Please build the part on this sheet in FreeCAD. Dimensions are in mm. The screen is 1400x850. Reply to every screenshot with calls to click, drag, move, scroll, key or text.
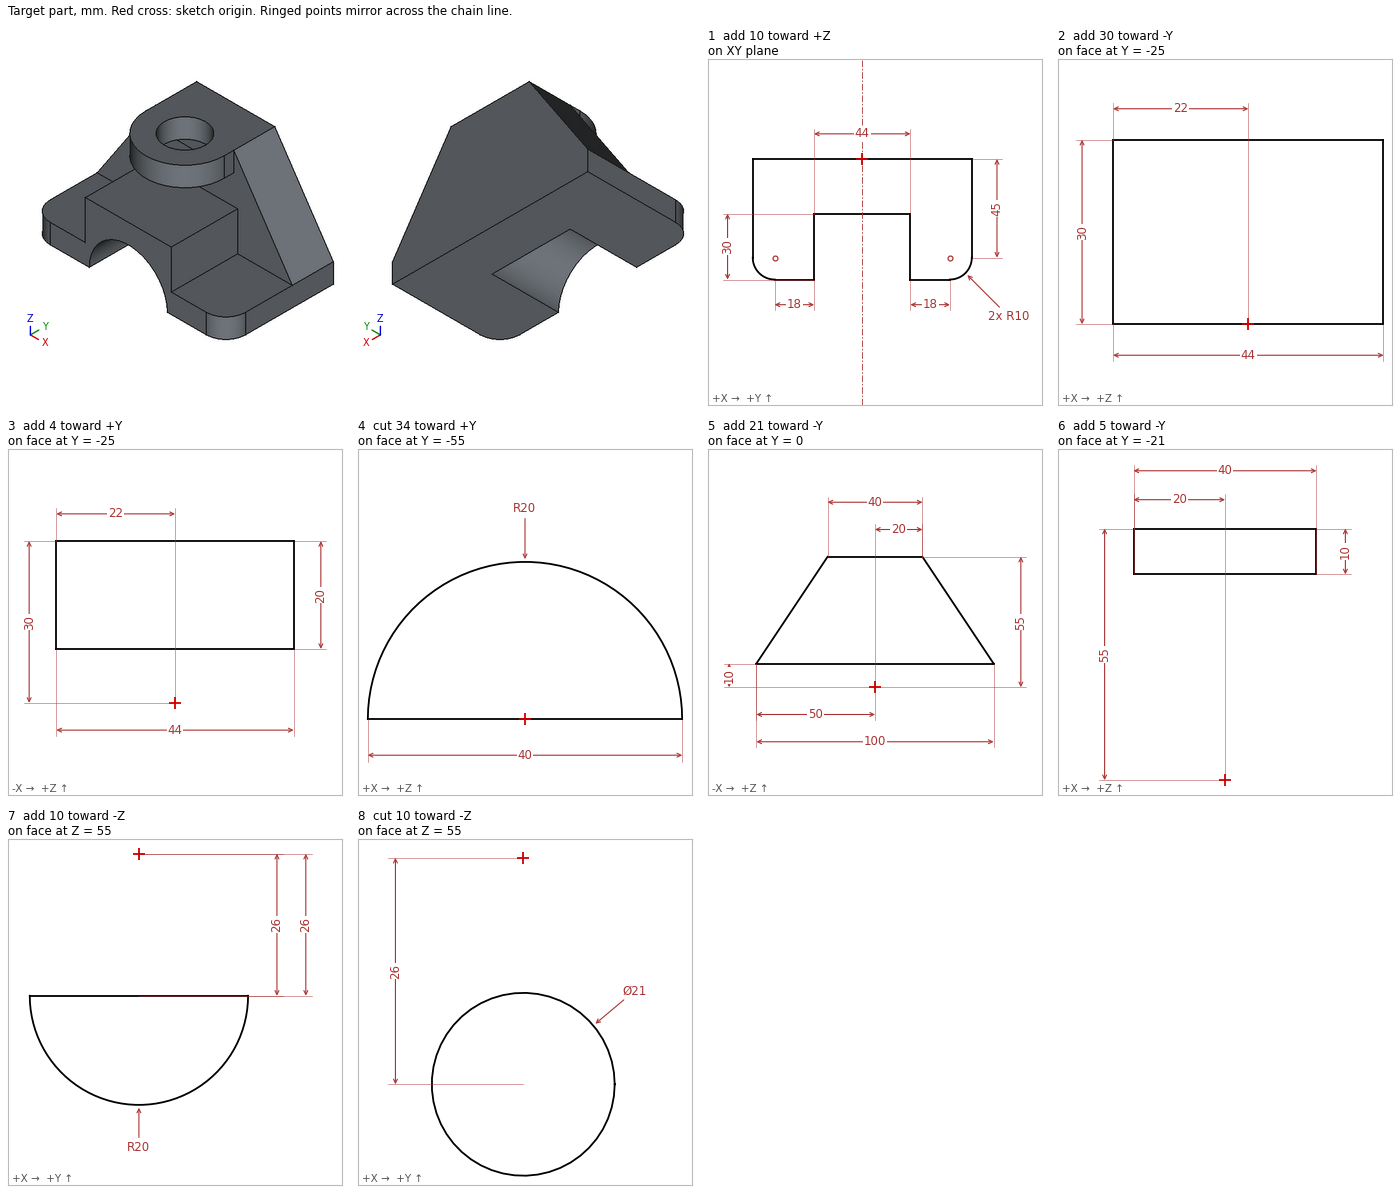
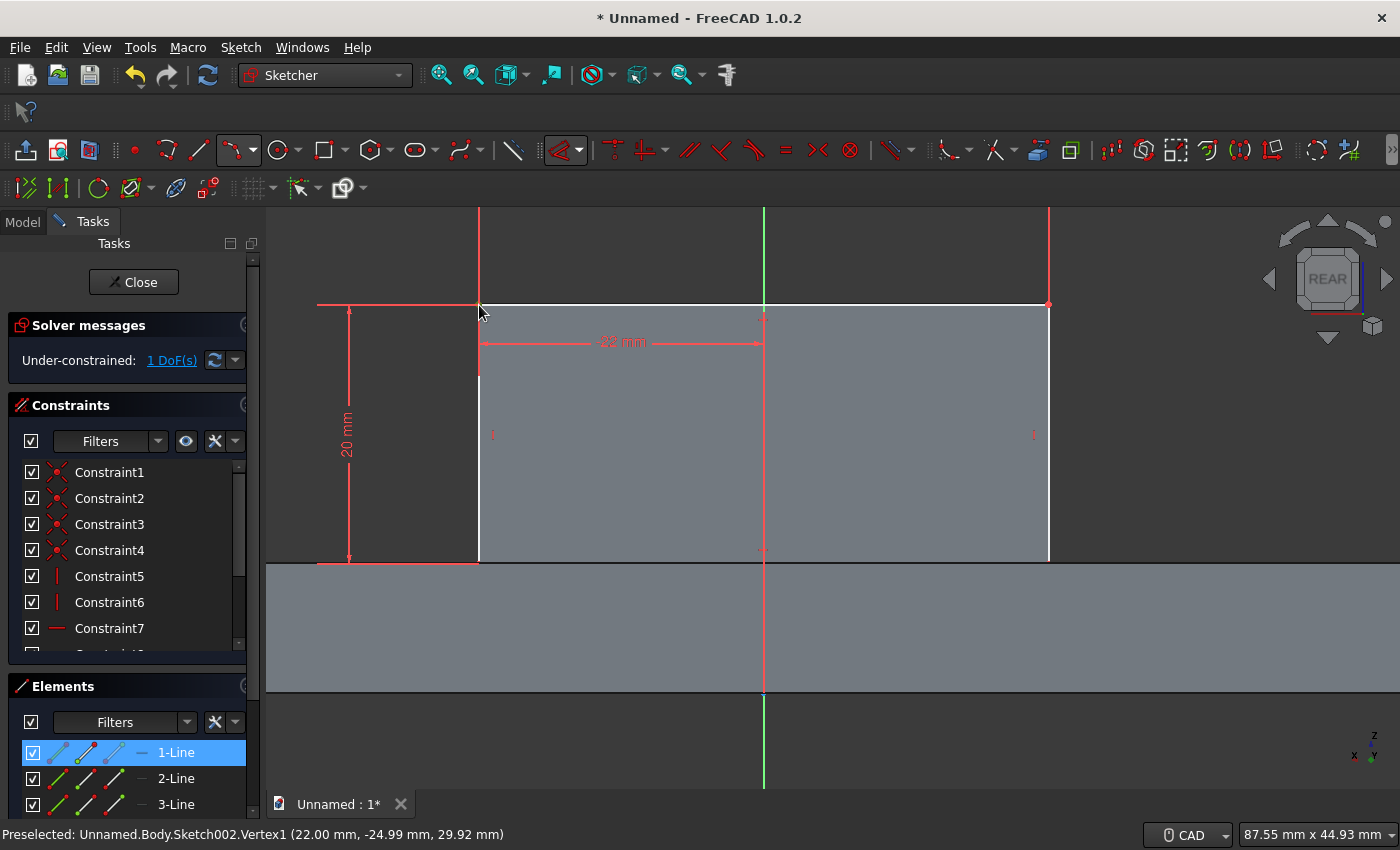
click(582, 150)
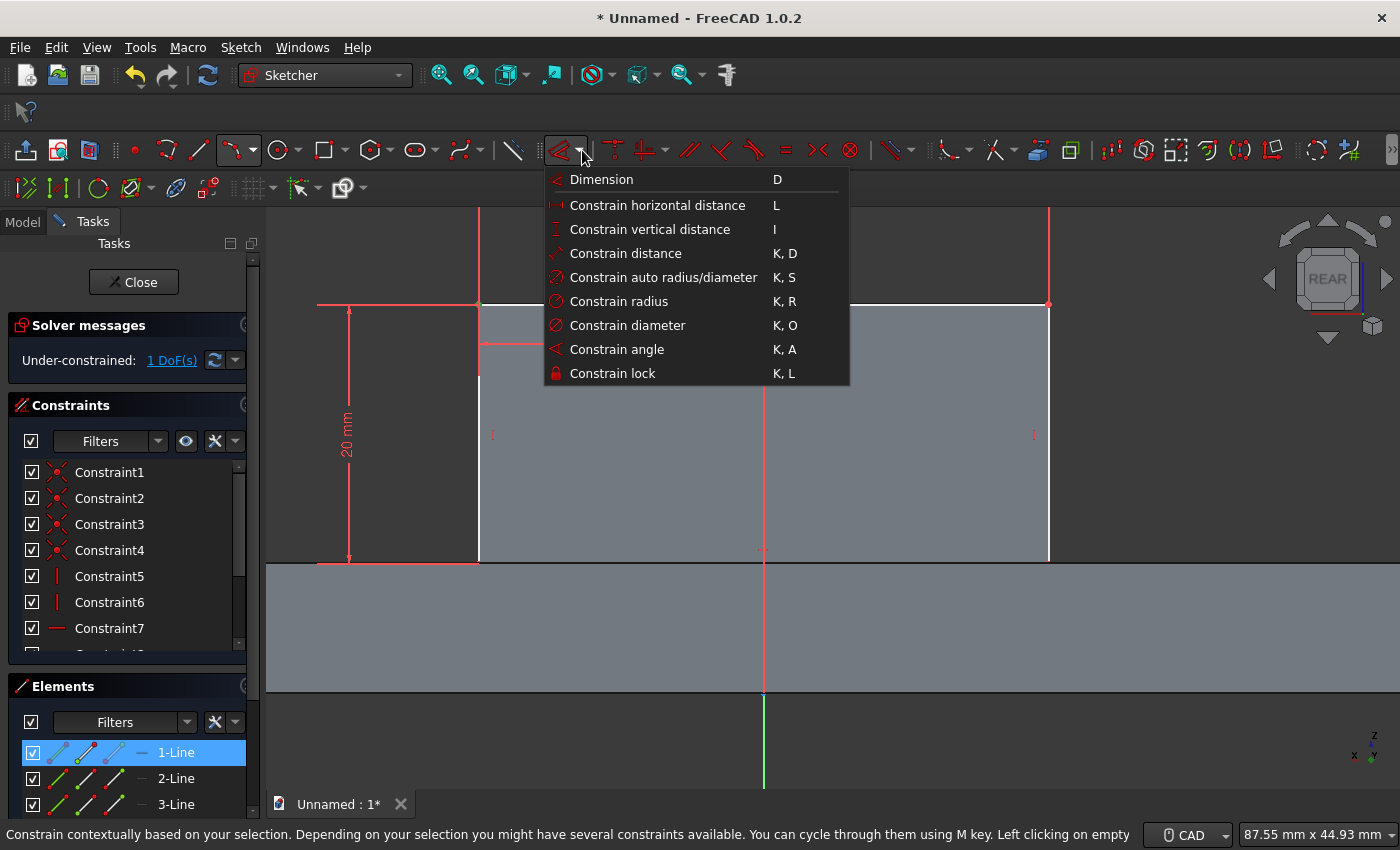
click(697, 229)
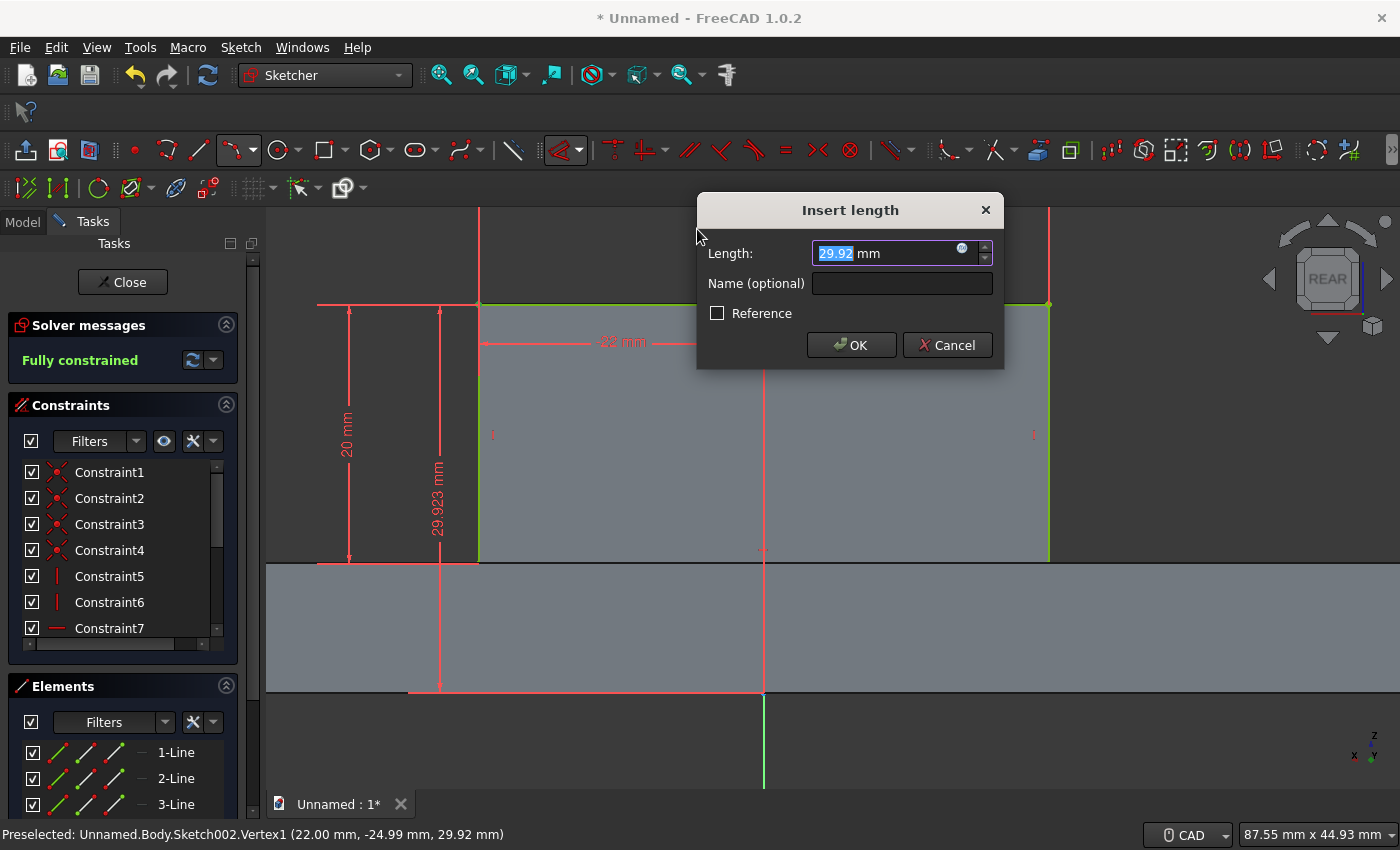
text(30)
key(Return)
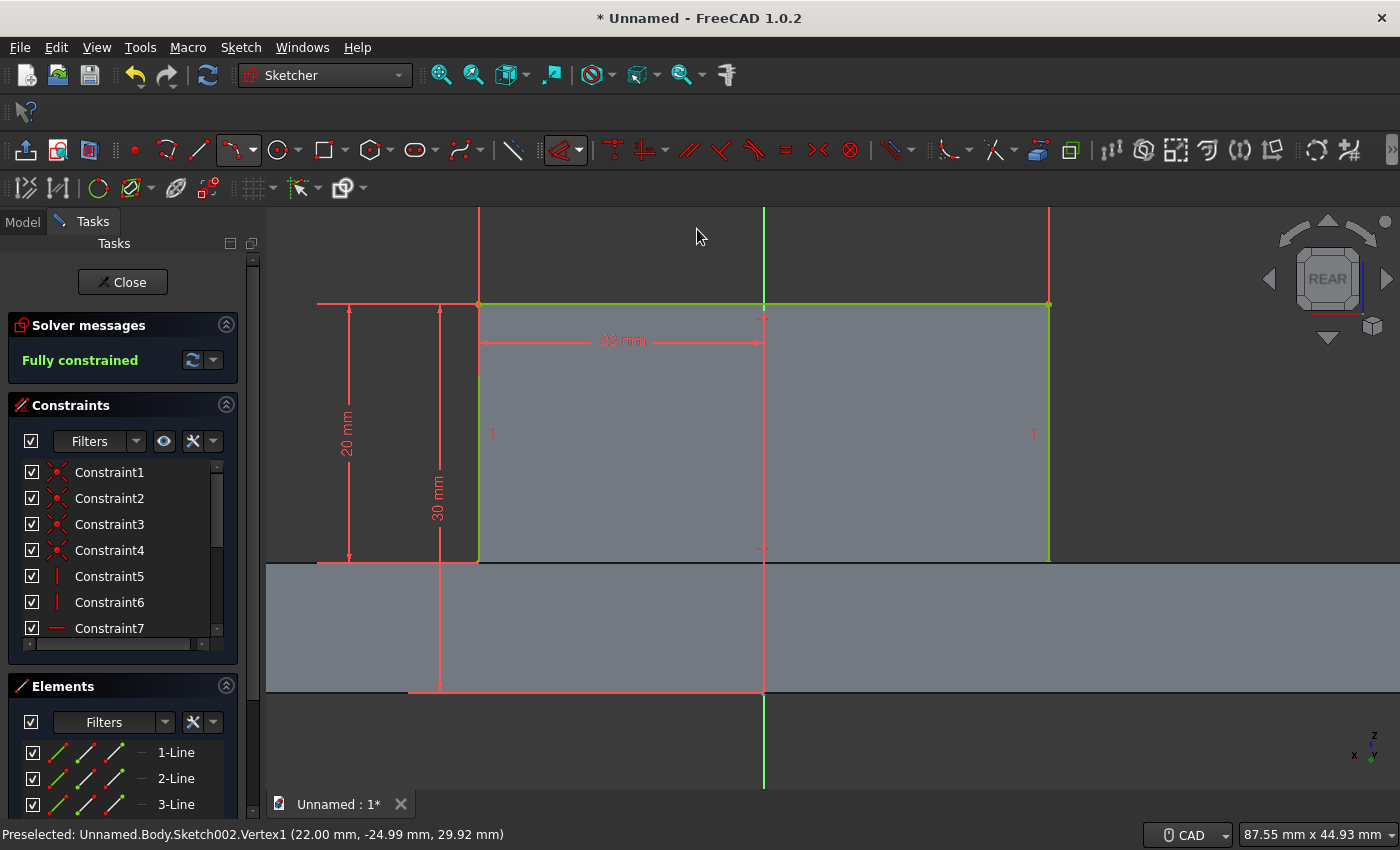
click(123, 282)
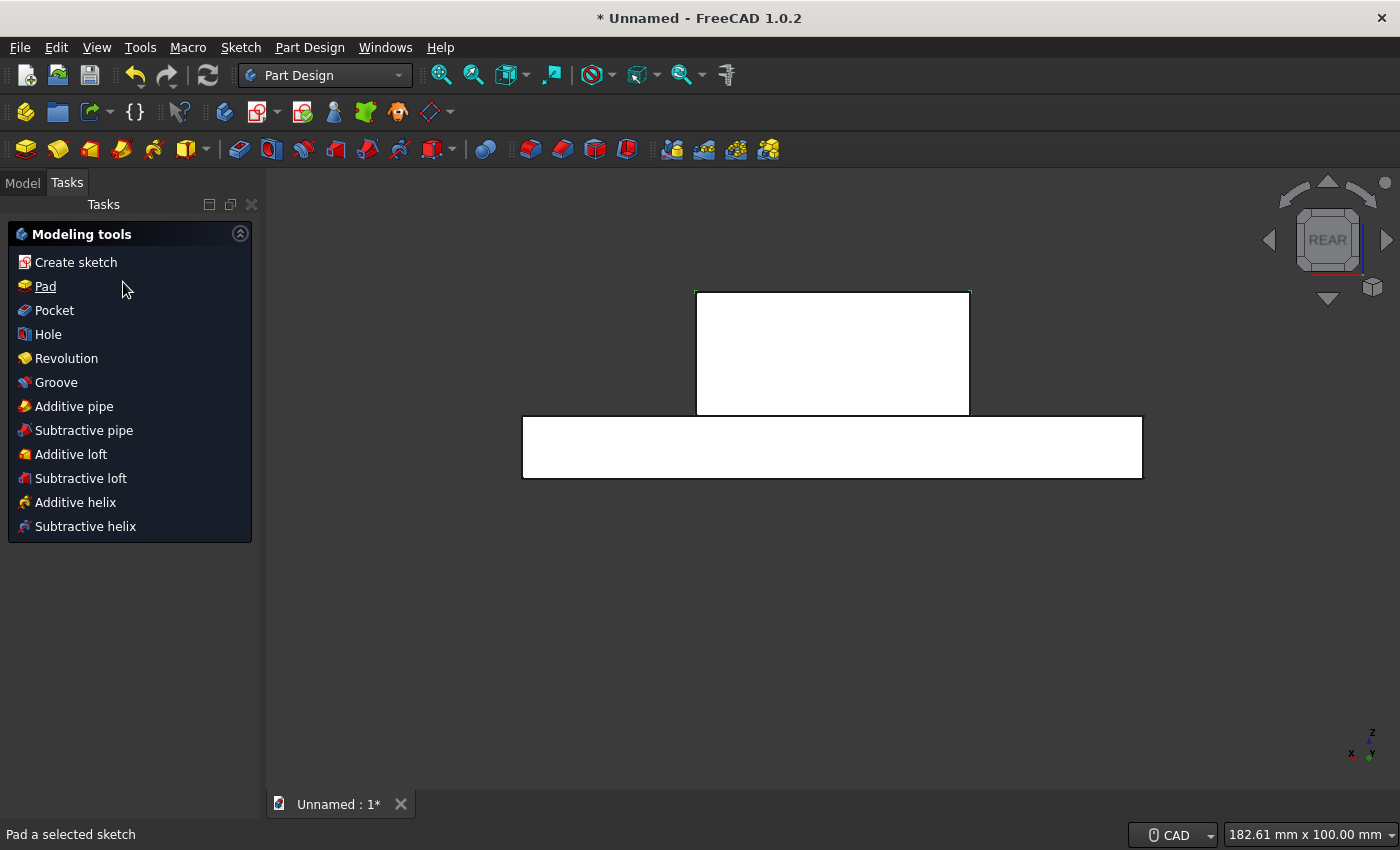
click(26, 150)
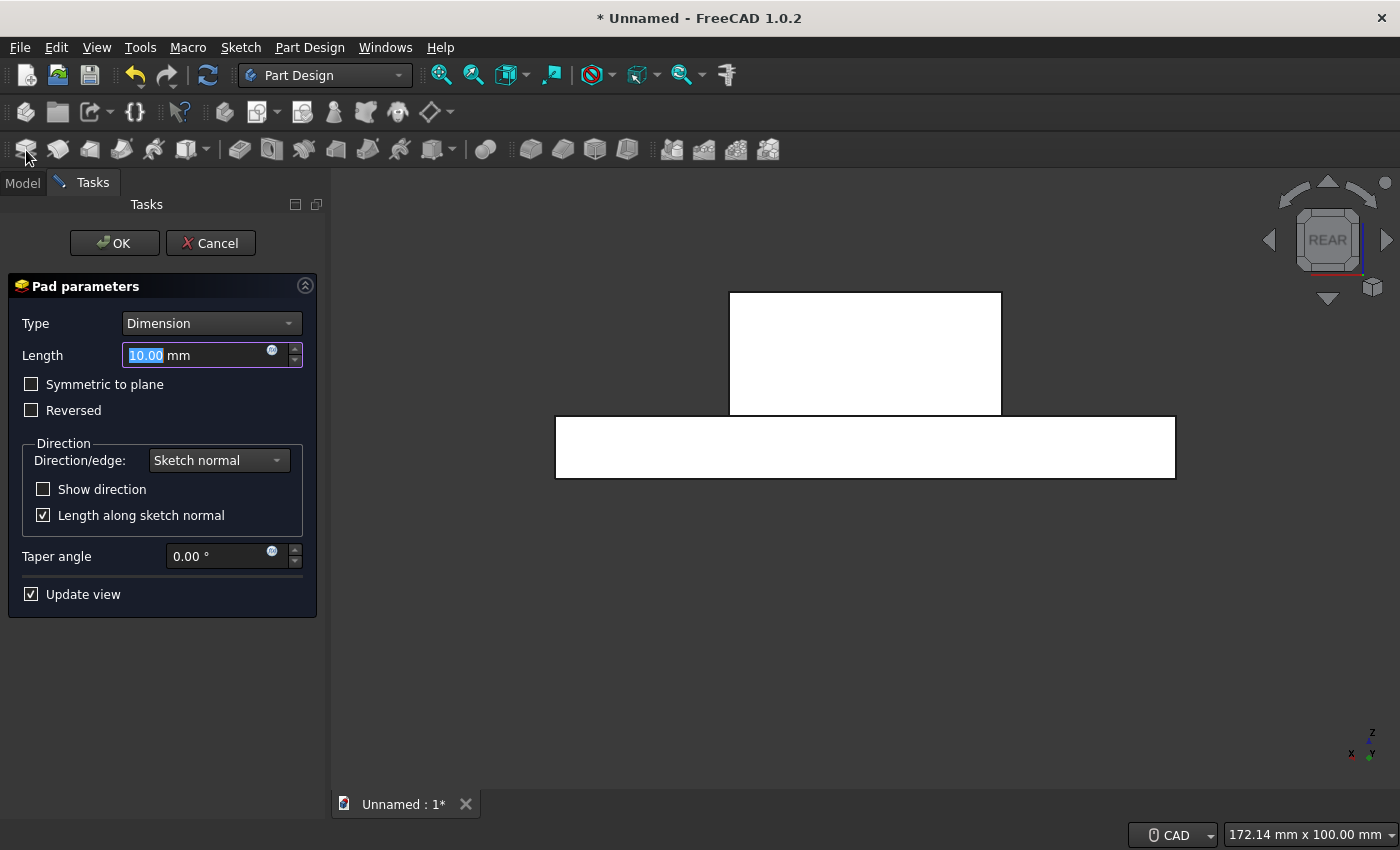
text(4)
key(Tab)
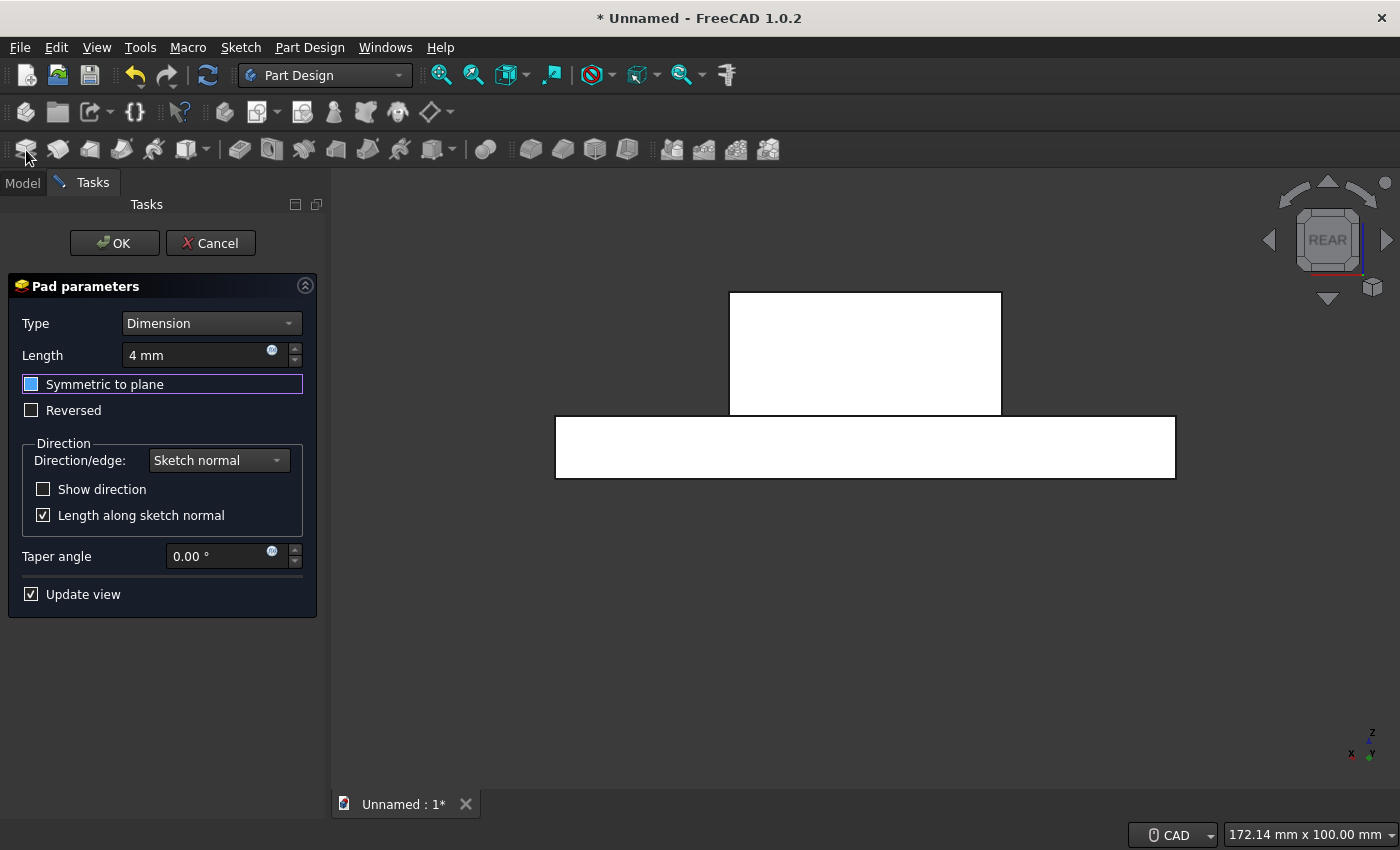
click(115, 243)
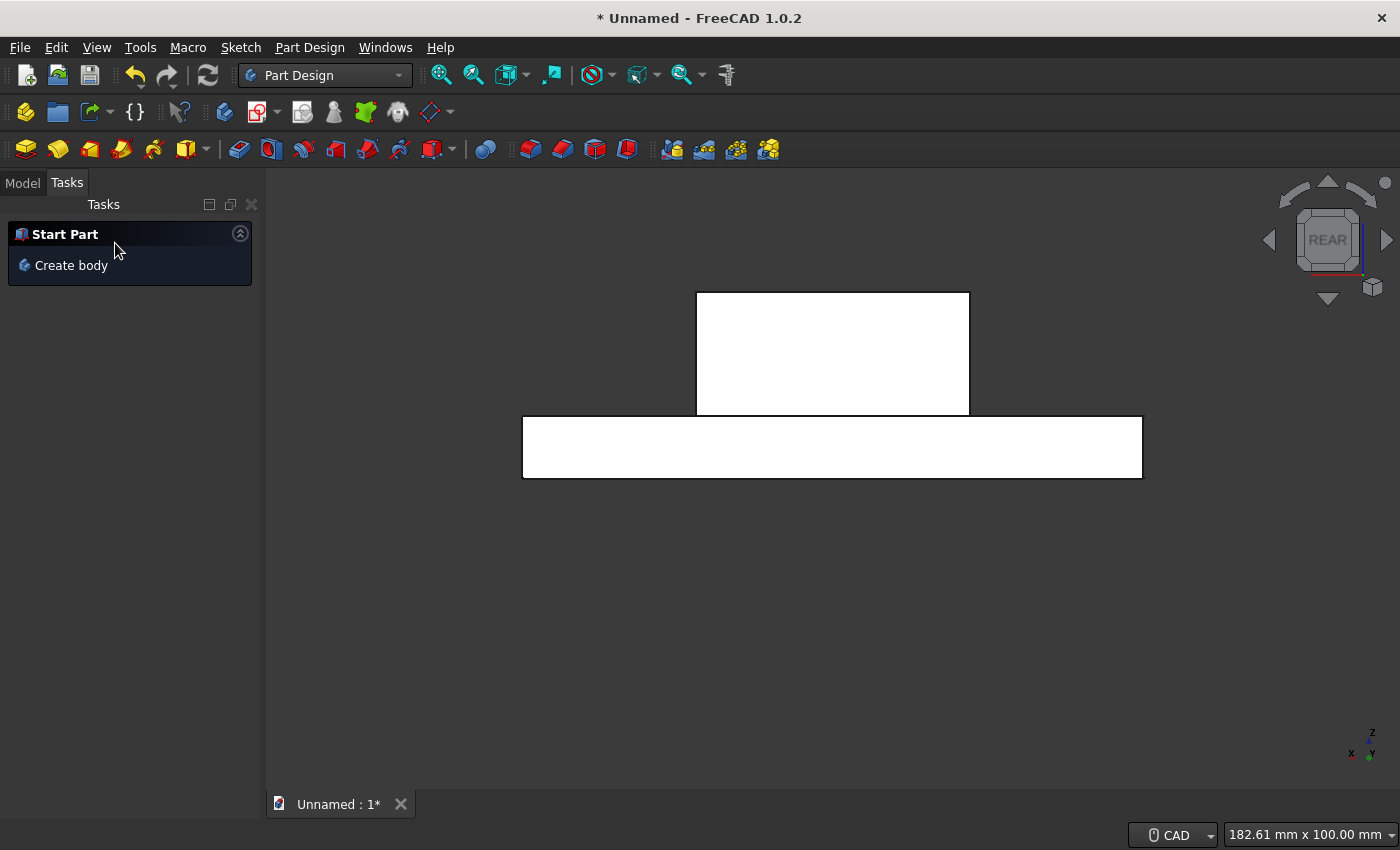
key(0)